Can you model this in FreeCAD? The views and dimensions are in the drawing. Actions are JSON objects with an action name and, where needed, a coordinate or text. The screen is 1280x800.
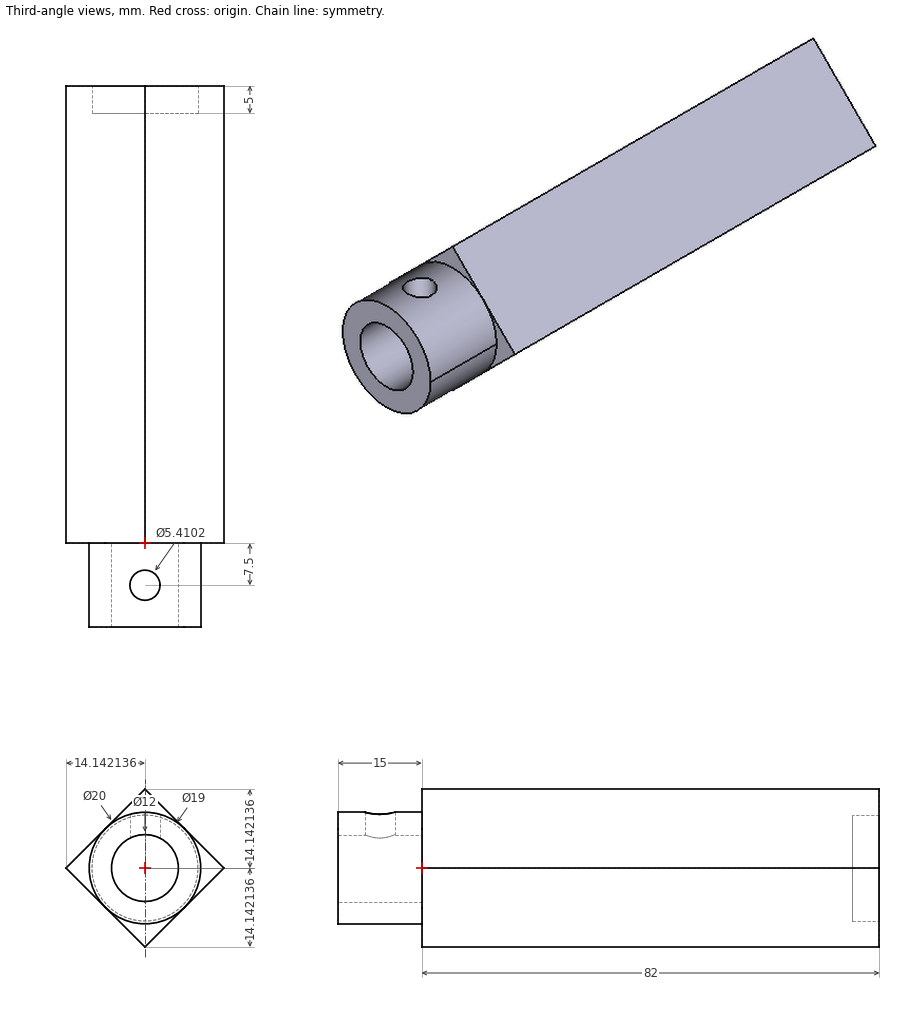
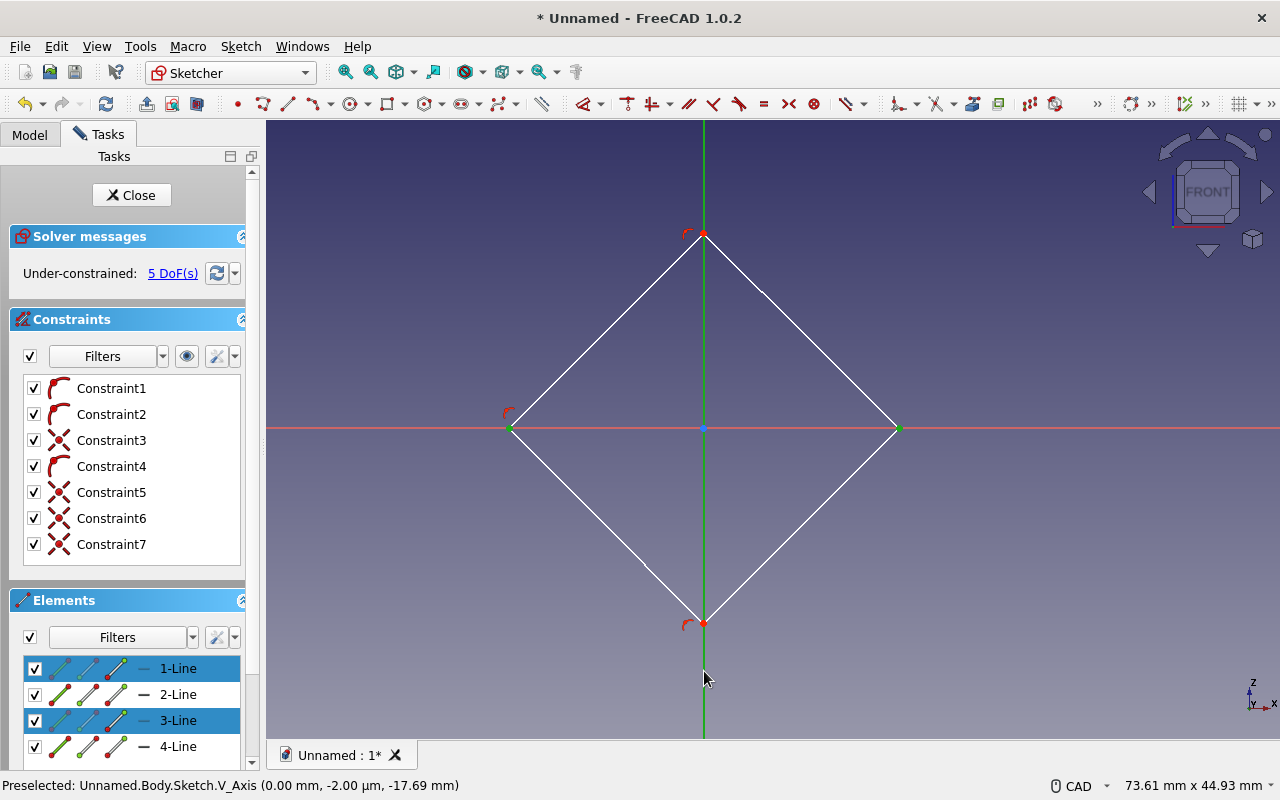
{"action": "left_click", "coordinate": [789, 104]}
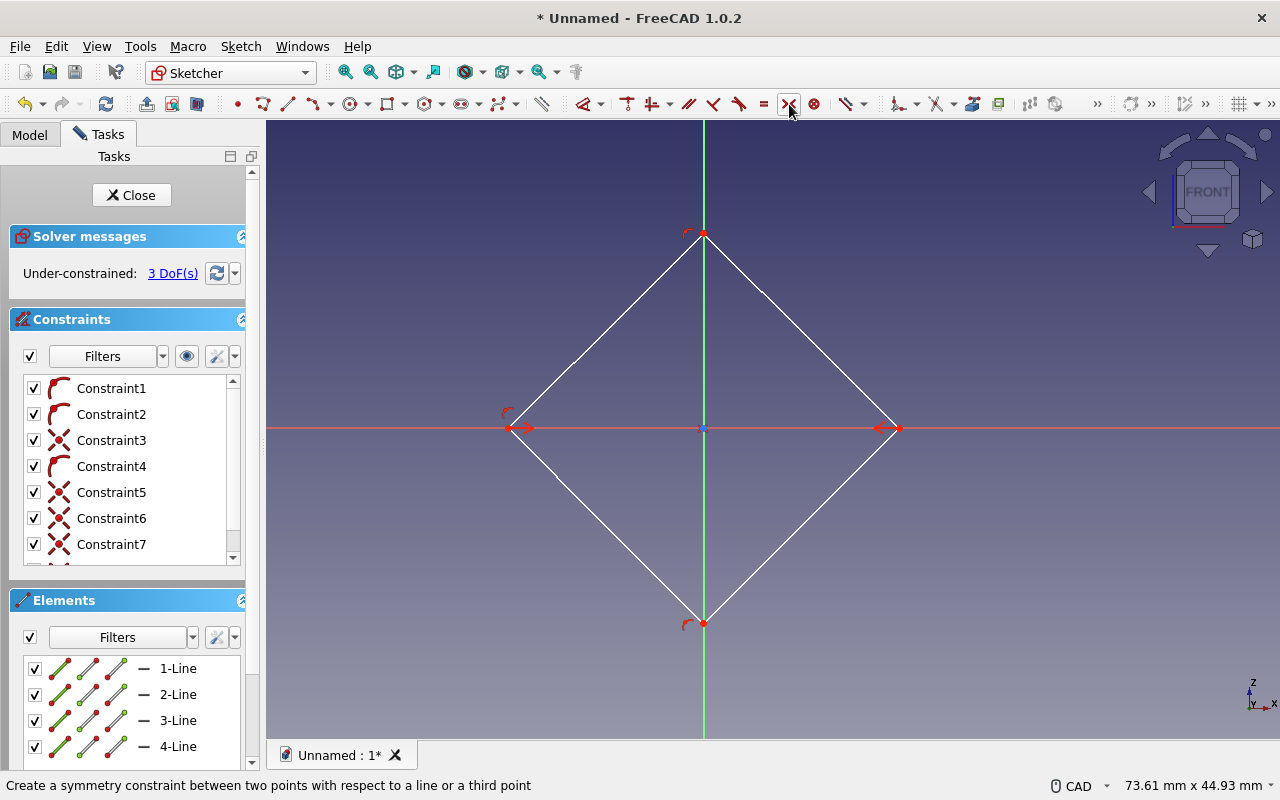
{"action": "left_click", "coordinate": [582, 104]}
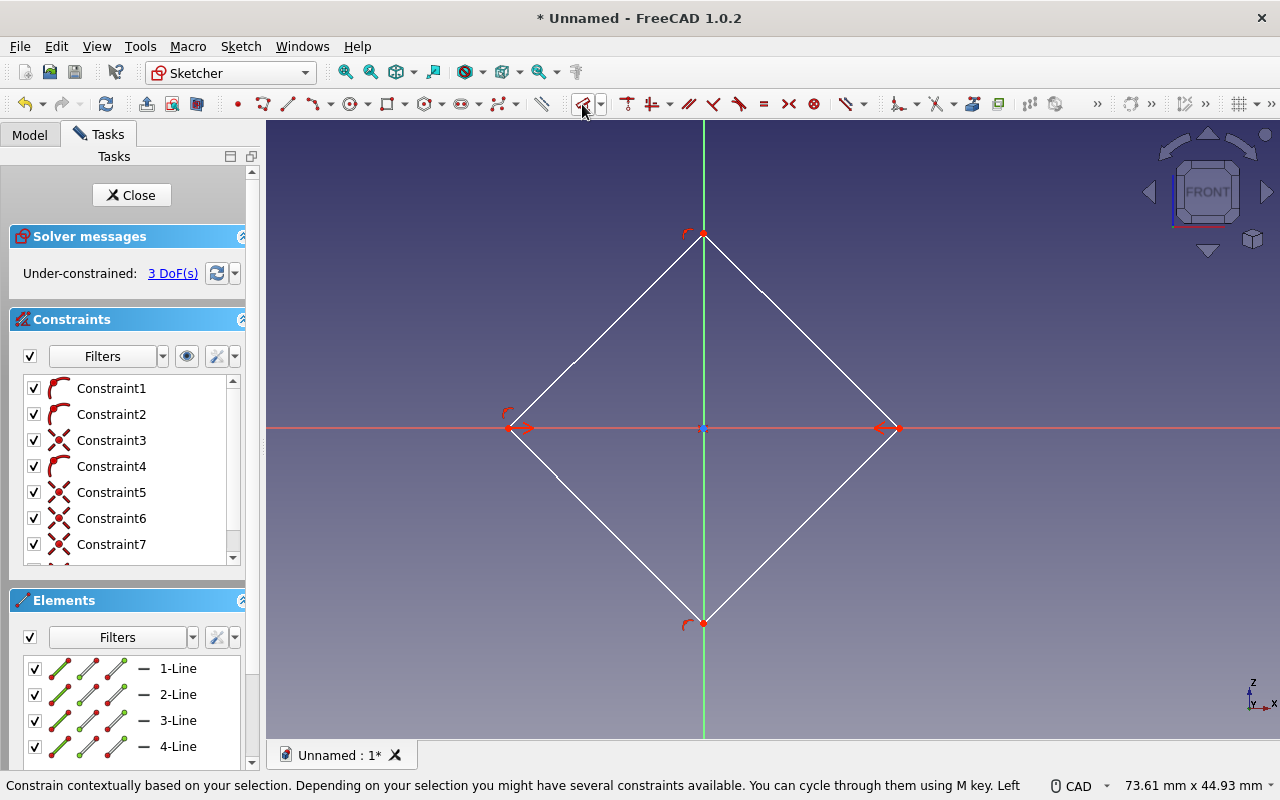
{"action": "left_click", "coordinate": [704, 624]}
{"action": "left_click", "coordinate": [738, 526]}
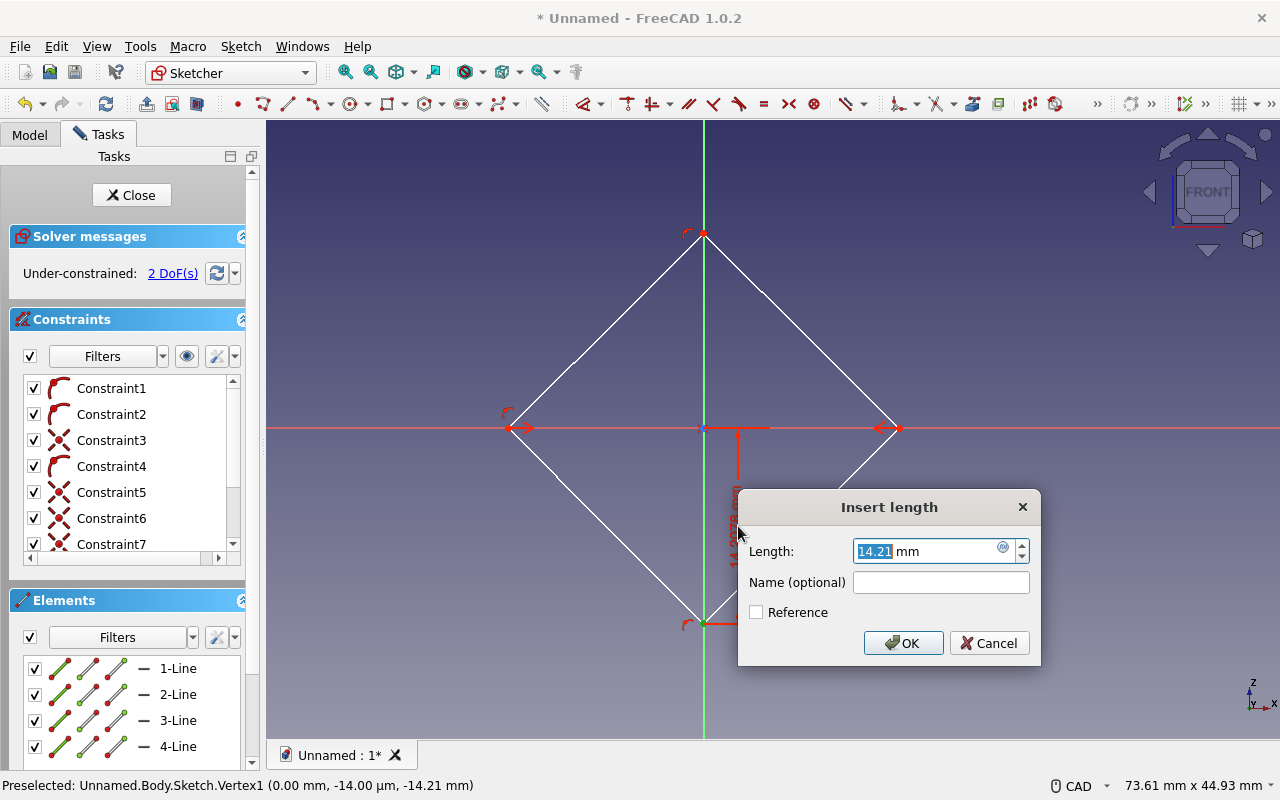
{"action": "type", "text": "14.142136"}
{"action": "key", "text": "Return"}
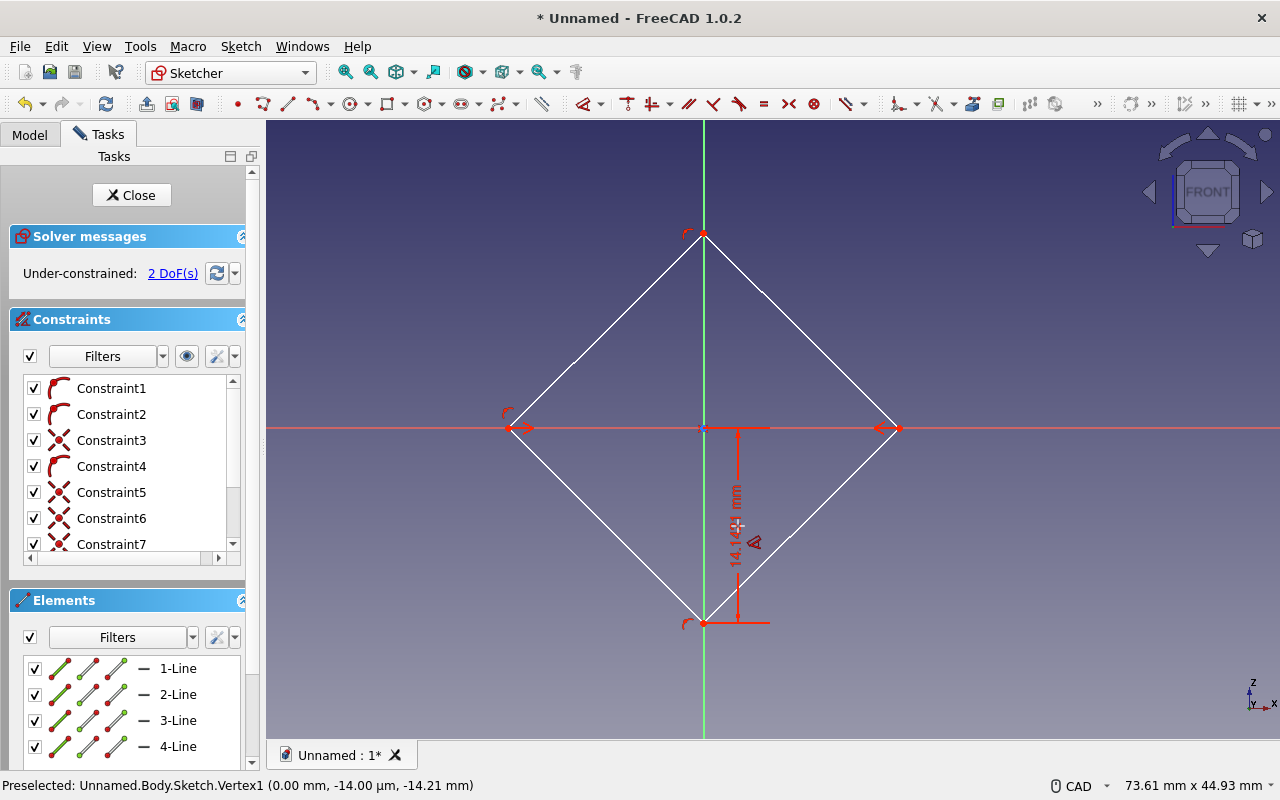
{"action": "left_click", "coordinate": [508, 428]}
{"action": "left_click", "coordinate": [606, 462]}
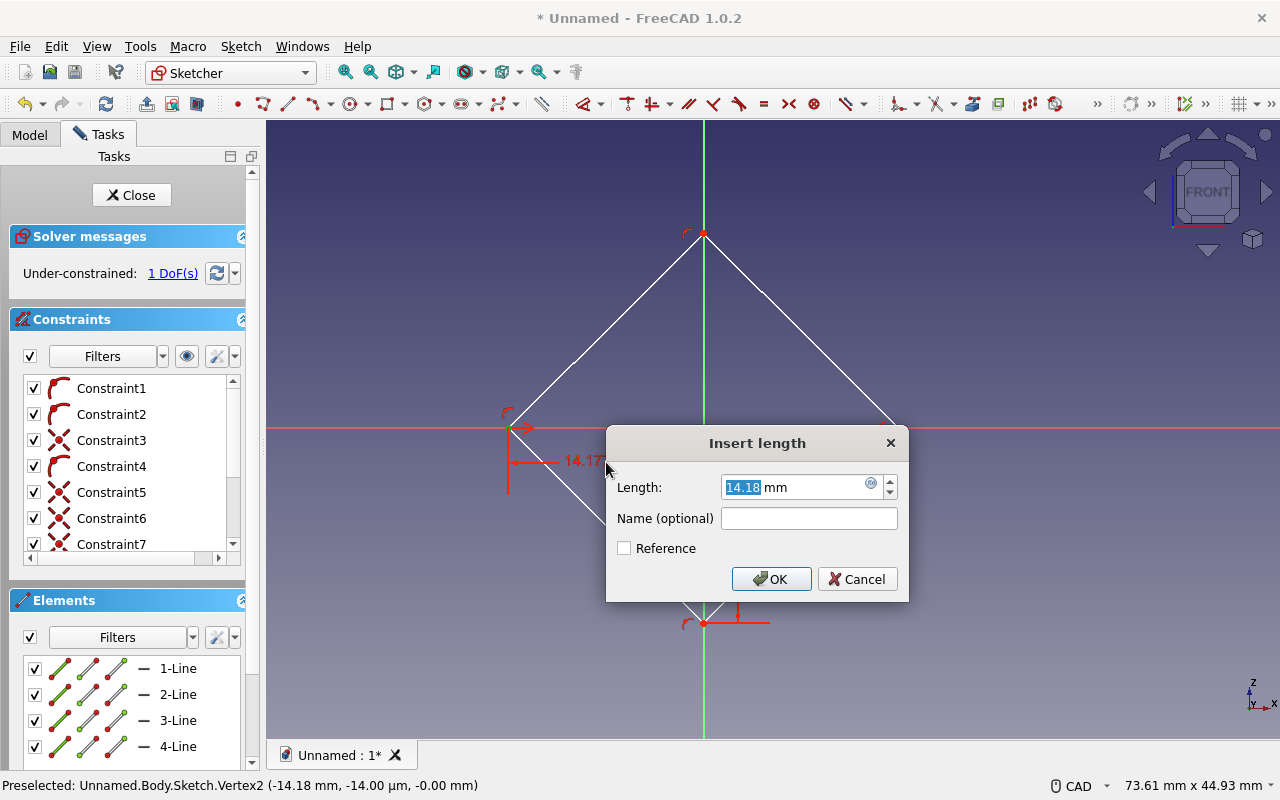
{"action": "type", "text": "14.142136"}
{"action": "key", "text": "Return"}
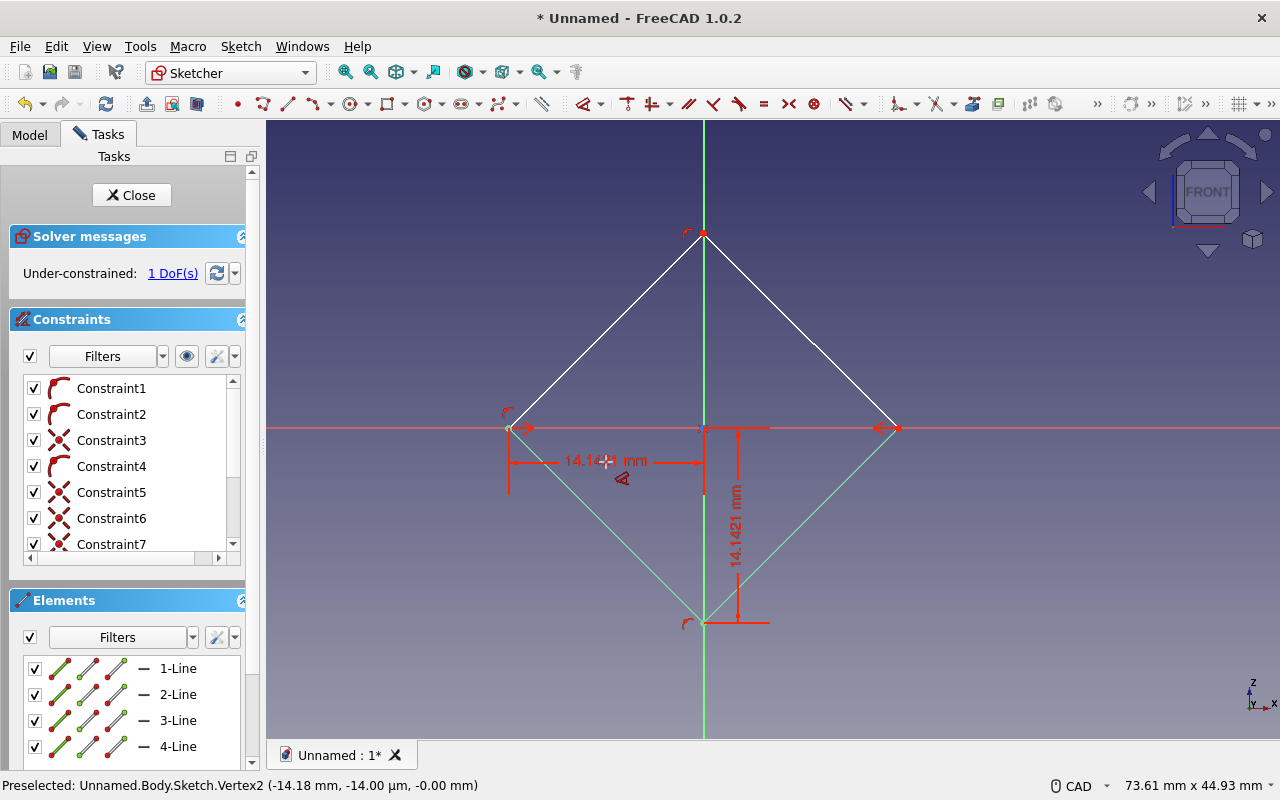
{"action": "left_click", "coordinate": [704, 234]}
{"action": "left_click", "coordinate": [738, 331]}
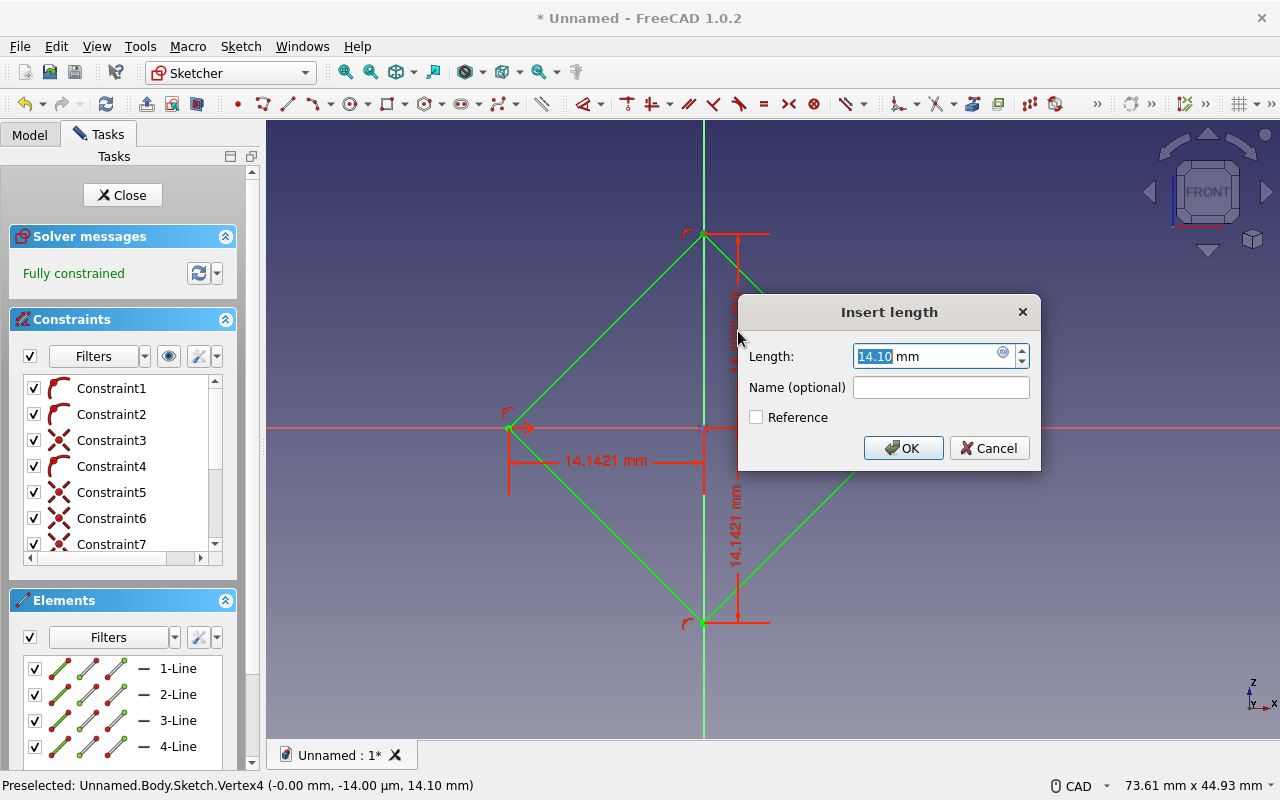
{"action": "type", "text": "14.142136"}
{"action": "key", "text": "Return"}
{"action": "key", "text": "Escape"}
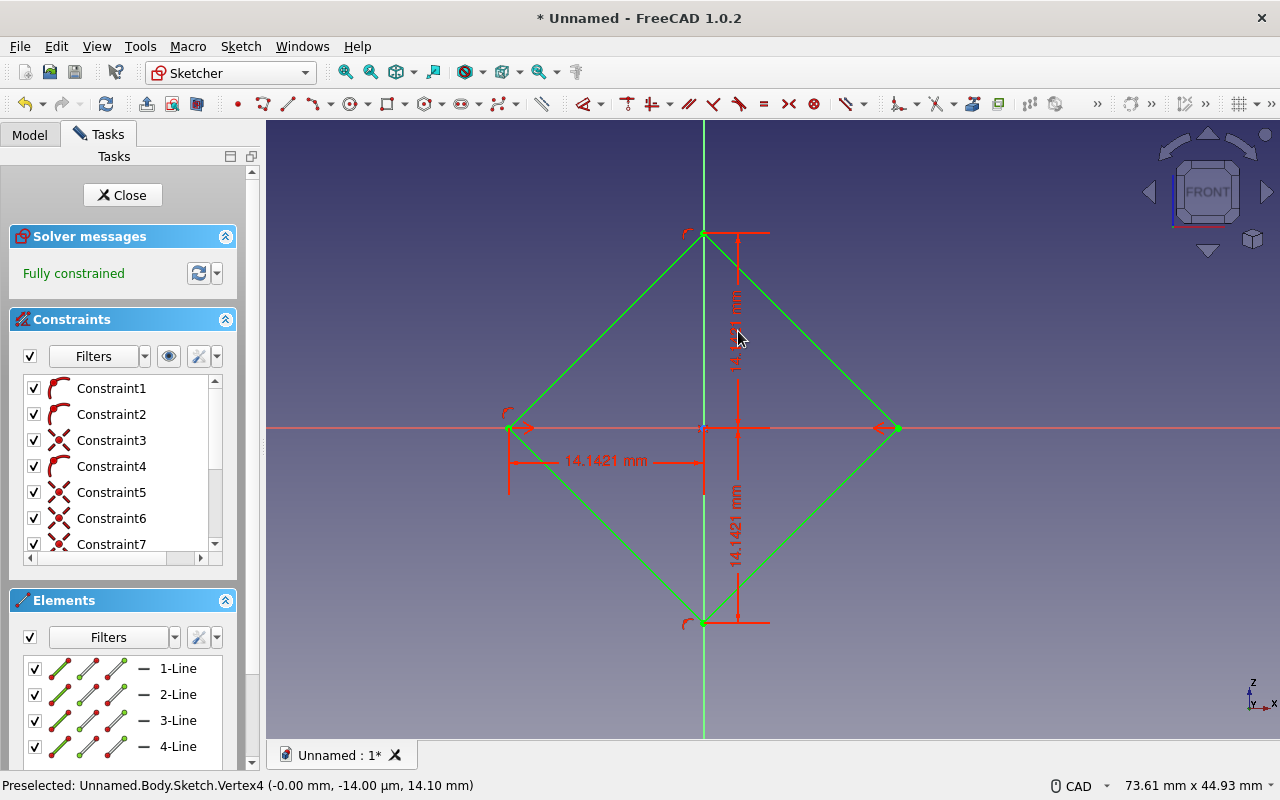
{"action": "left_click", "coordinate": [123, 195]}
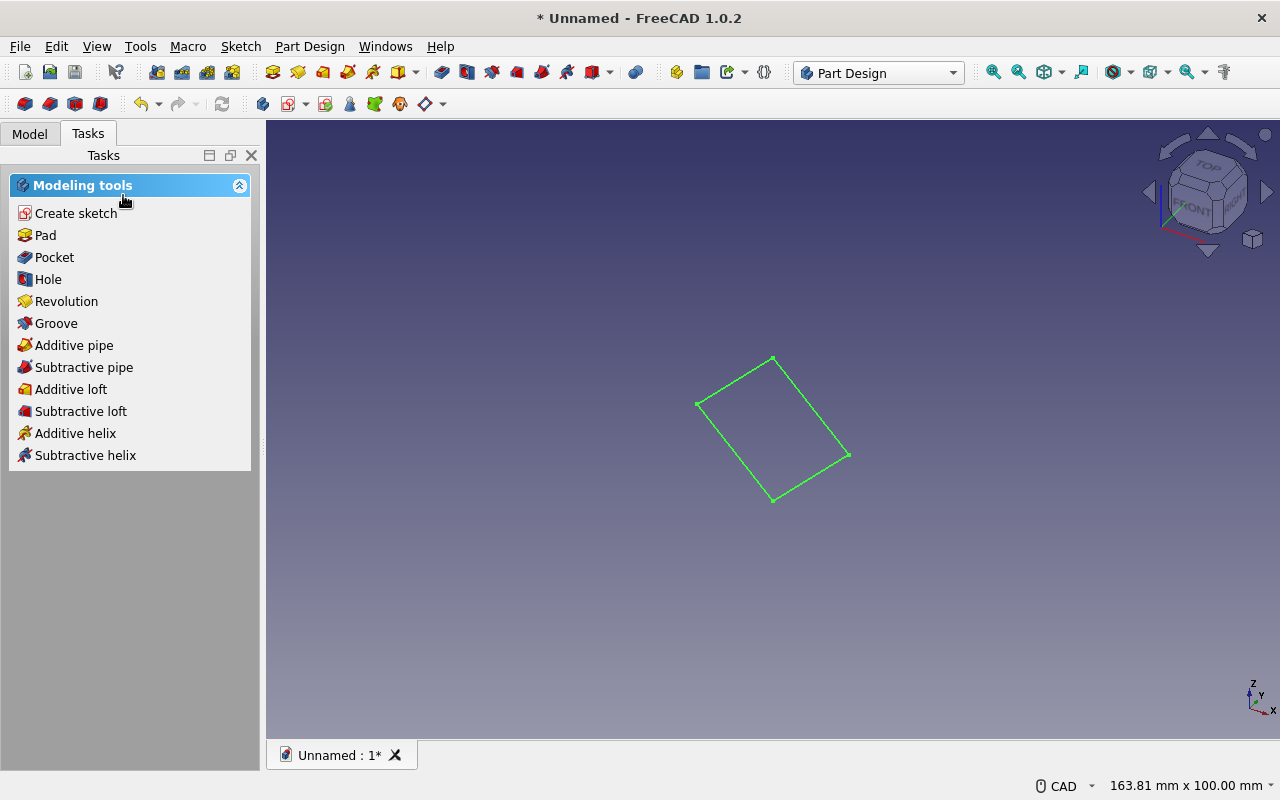
{"action": "left_click", "coordinate": [273, 72]}